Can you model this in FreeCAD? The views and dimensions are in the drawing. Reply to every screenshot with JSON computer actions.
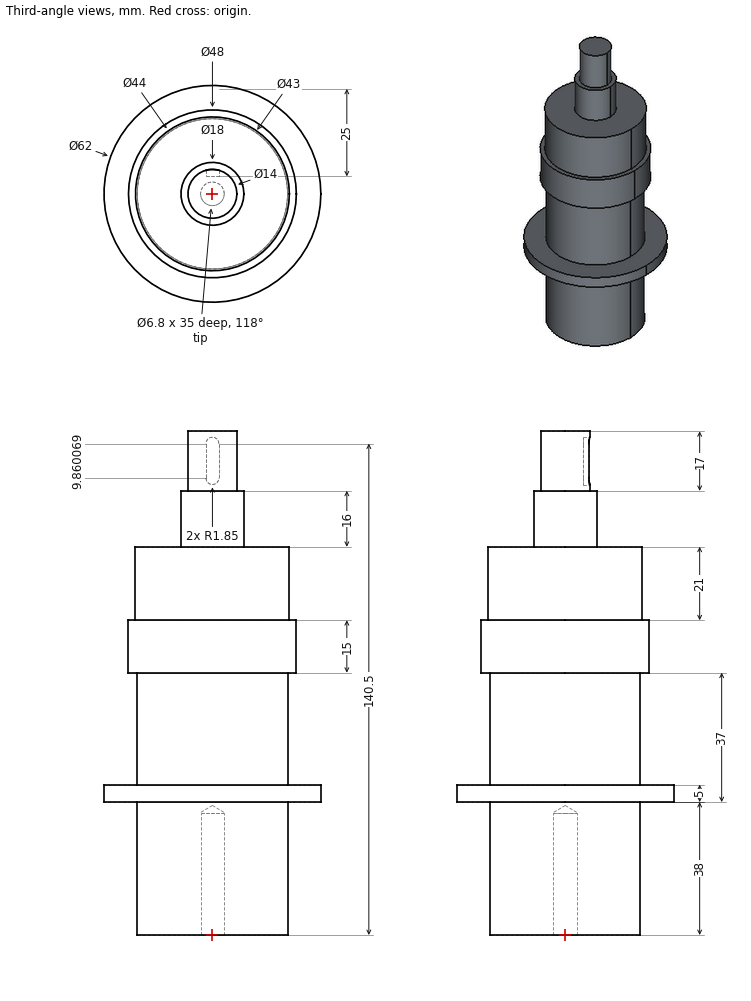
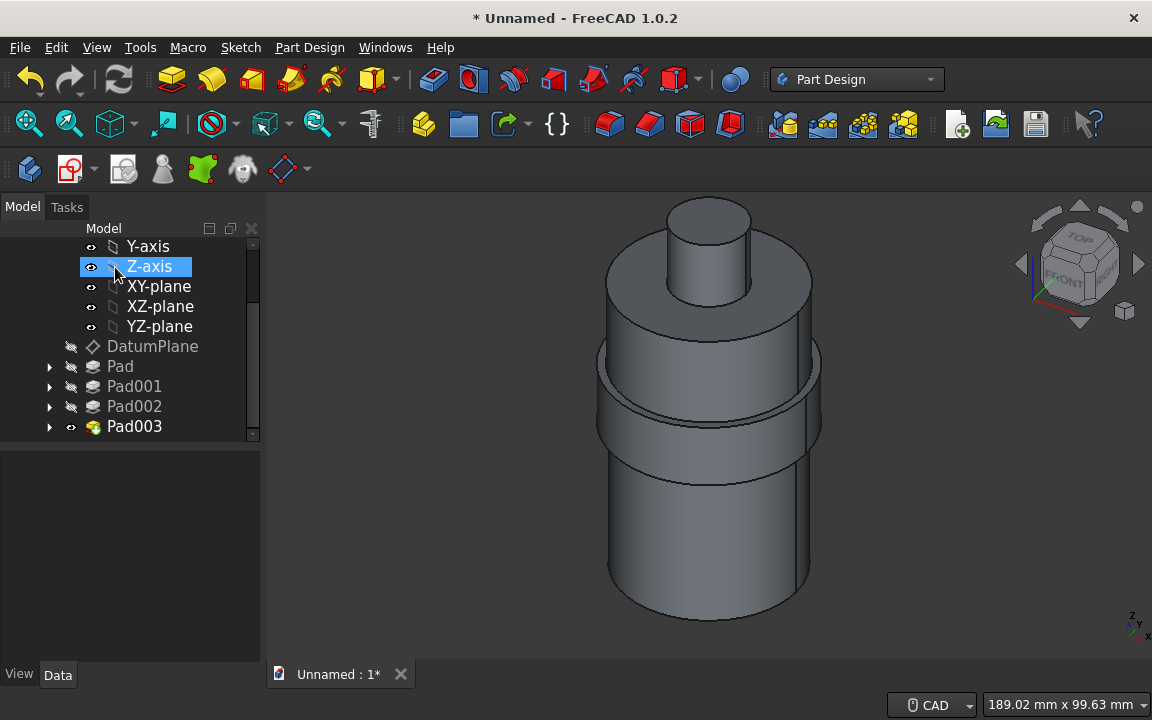
{"action": "left_click", "coordinate": [30, 124]}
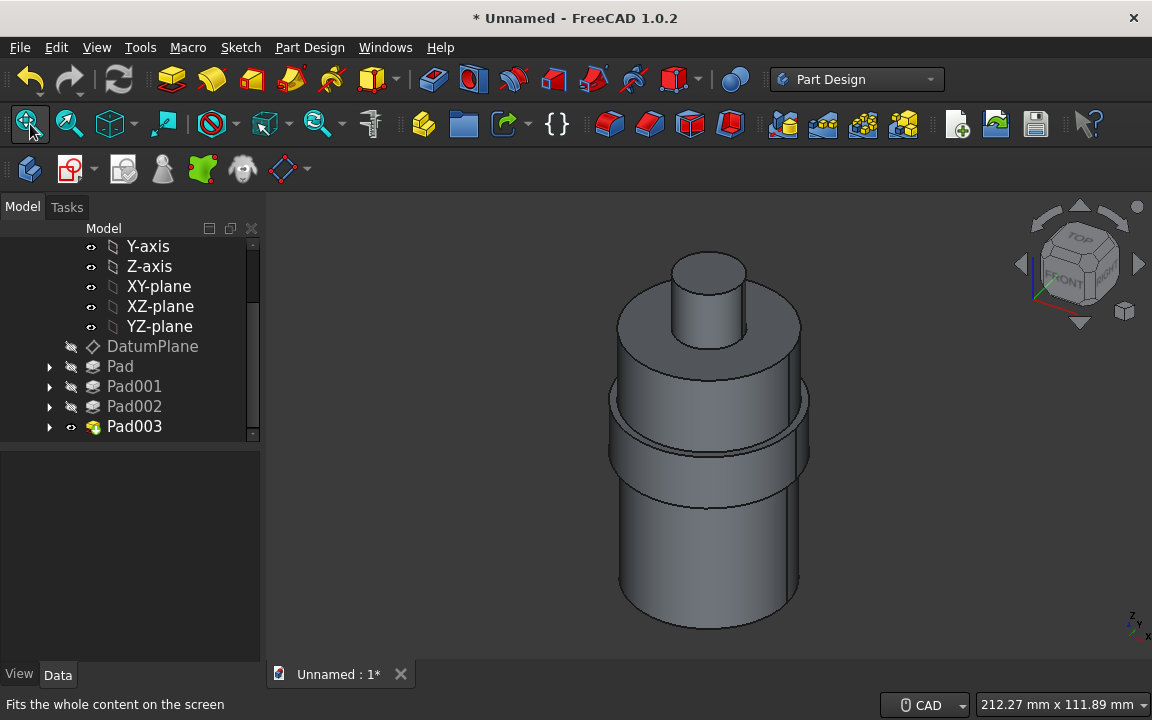
{"action": "left_click", "coordinate": [709, 272]}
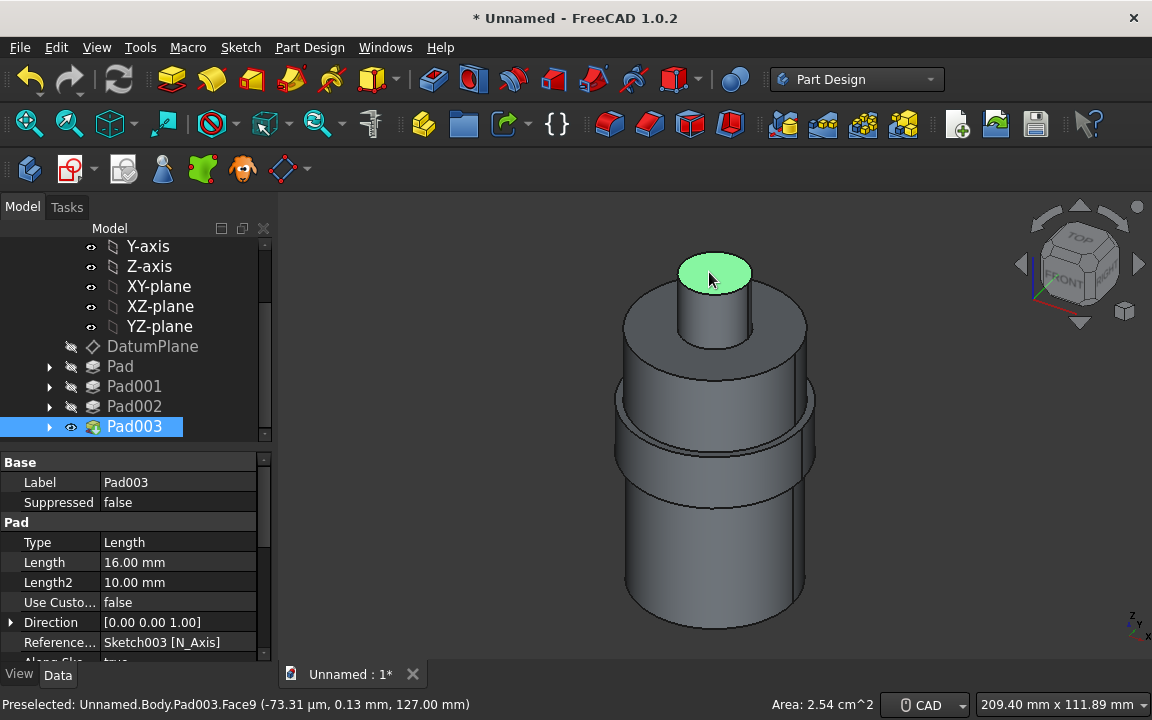
{"action": "left_click", "coordinate": [70, 170]}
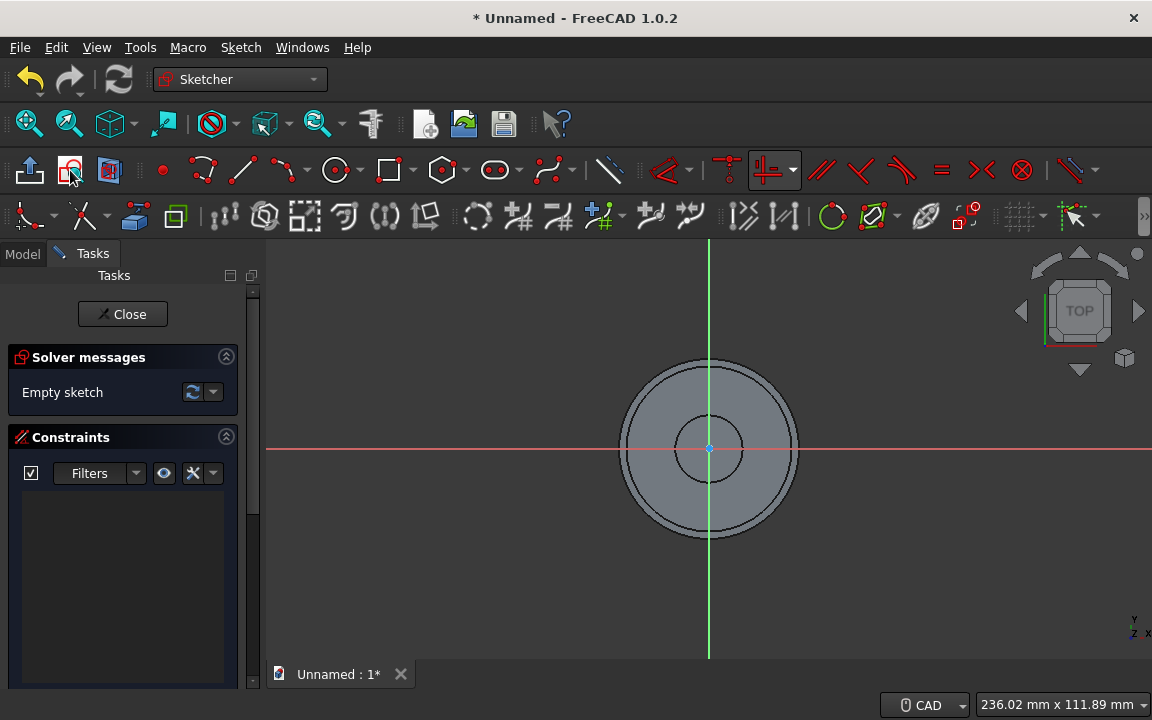
{"action": "scroll", "coordinate": [726, 449], "scroll_direction": "up", "scroll_amount": 8}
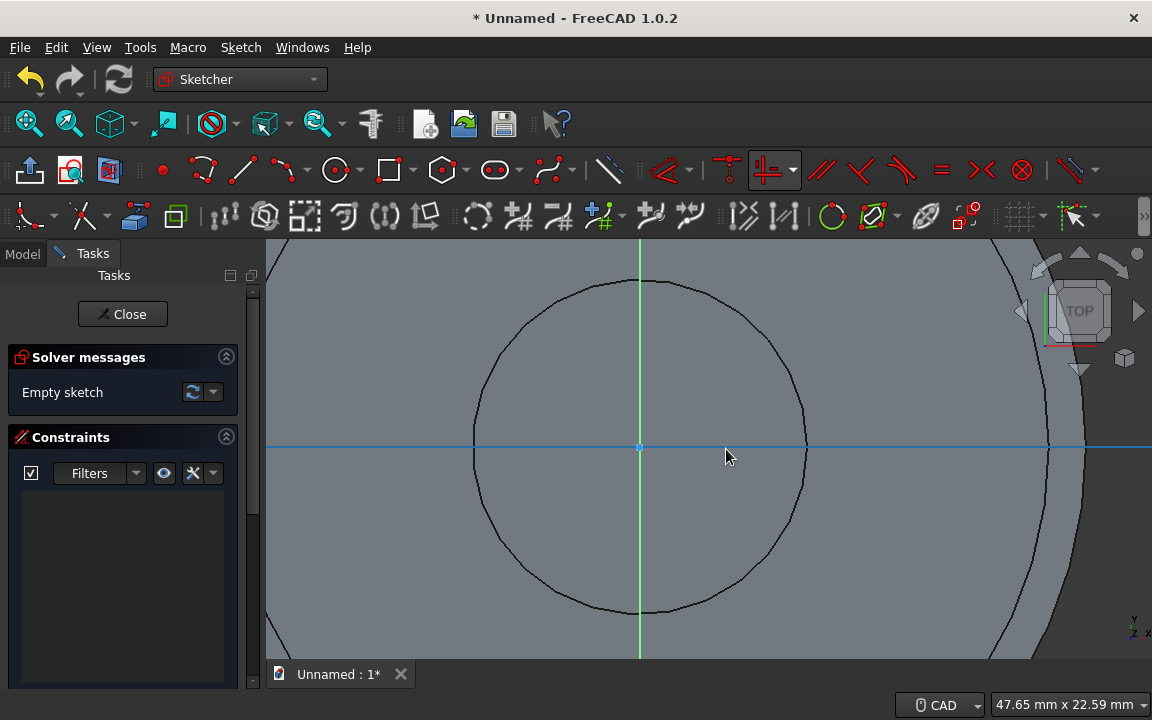
{"action": "key", "text": "g c"}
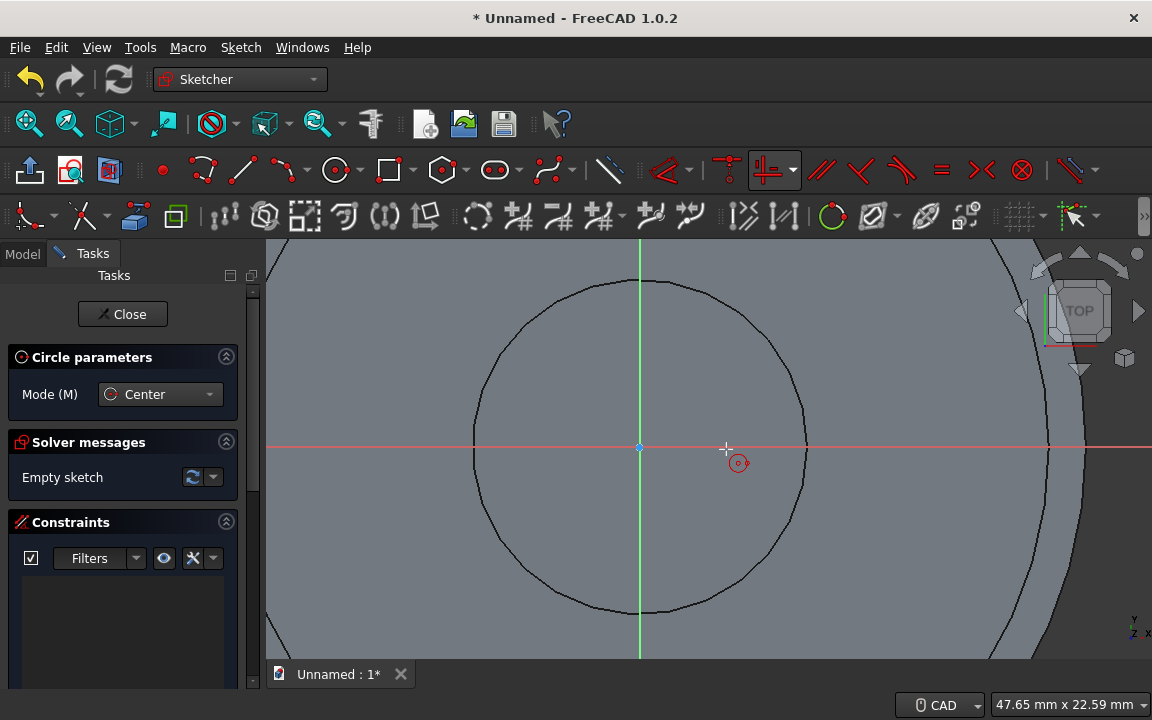
{"action": "left_click", "coordinate": [640, 447]}
{"action": "left_click", "coordinate": [732, 355]}
{"action": "key", "text": "Escape"}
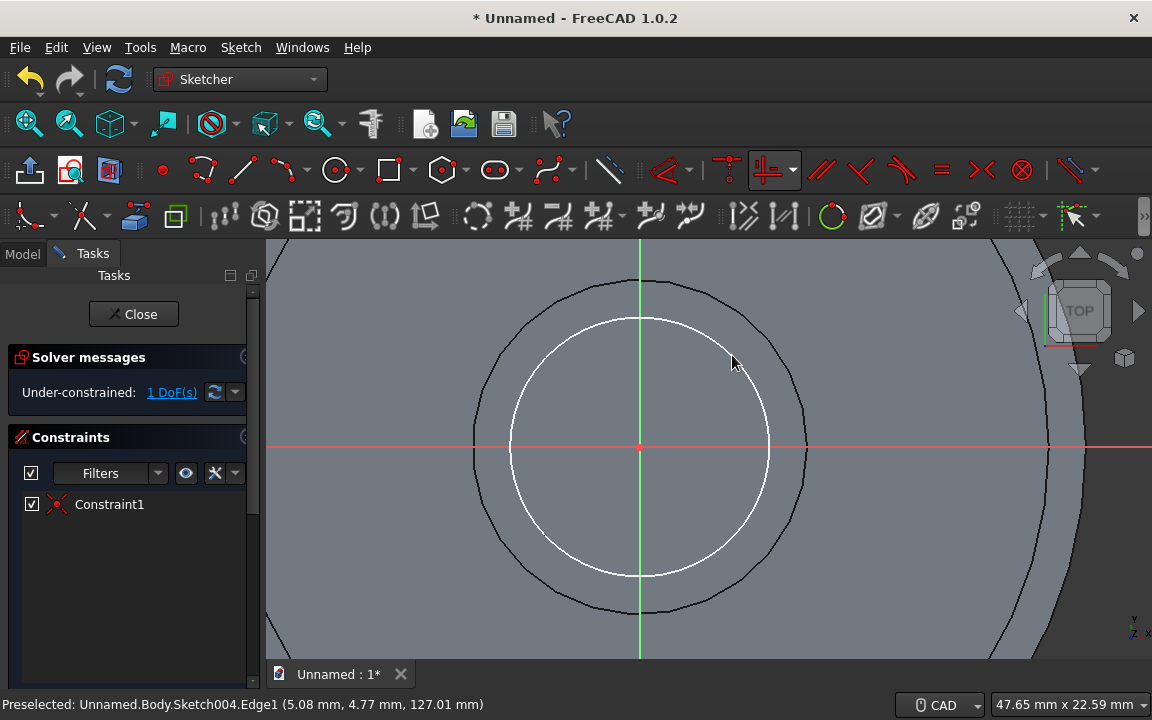
{"action": "left_click", "coordinate": [664, 170]}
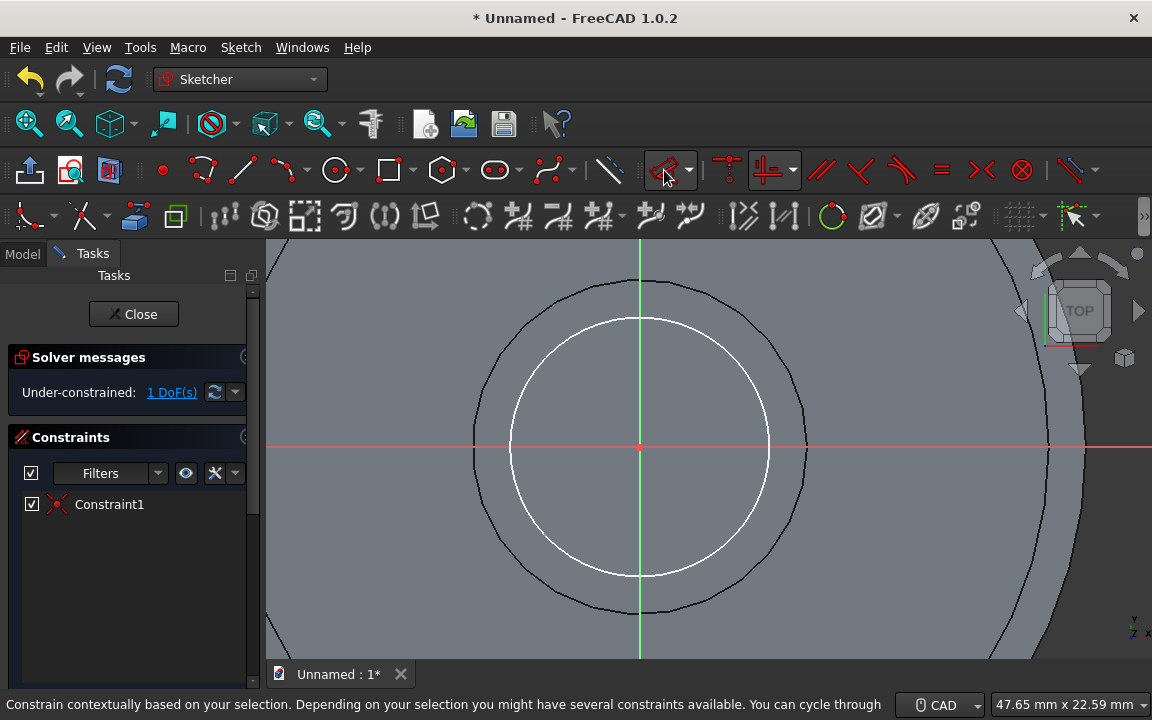
{"action": "left_click", "coordinate": [731, 355]}
{"action": "left_click", "coordinate": [754, 332]}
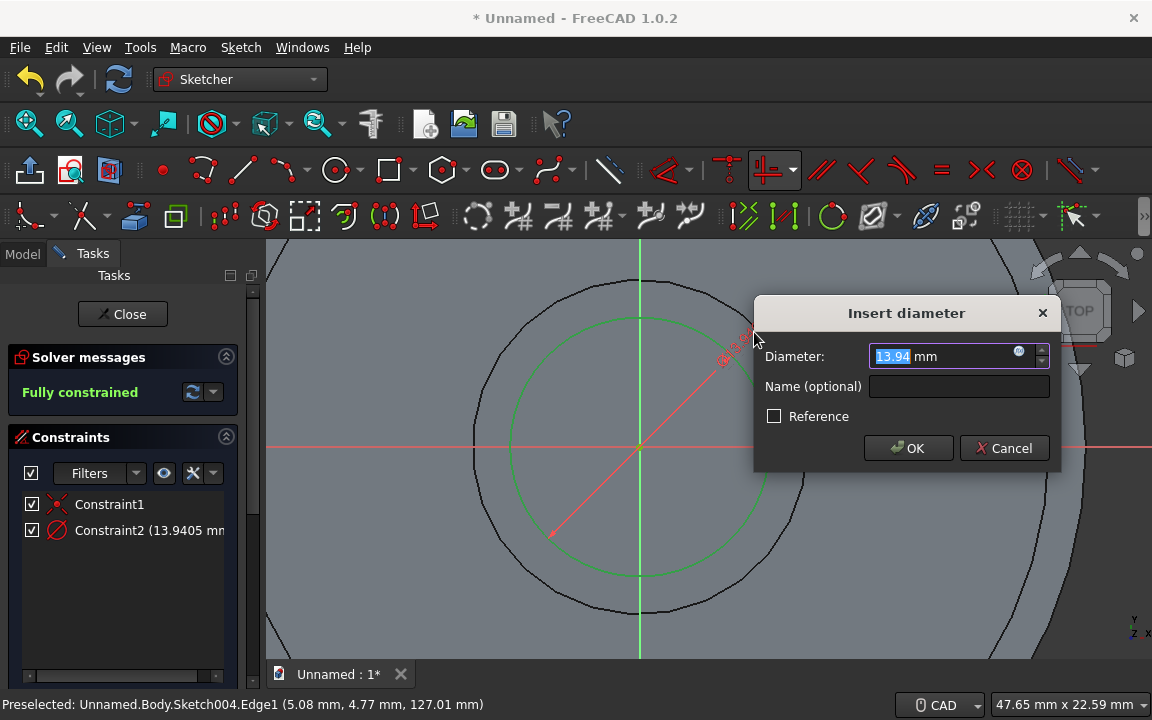
{"action": "type", "text": "14"}
{"action": "key", "text": "Return"}
{"action": "key", "text": "Escape"}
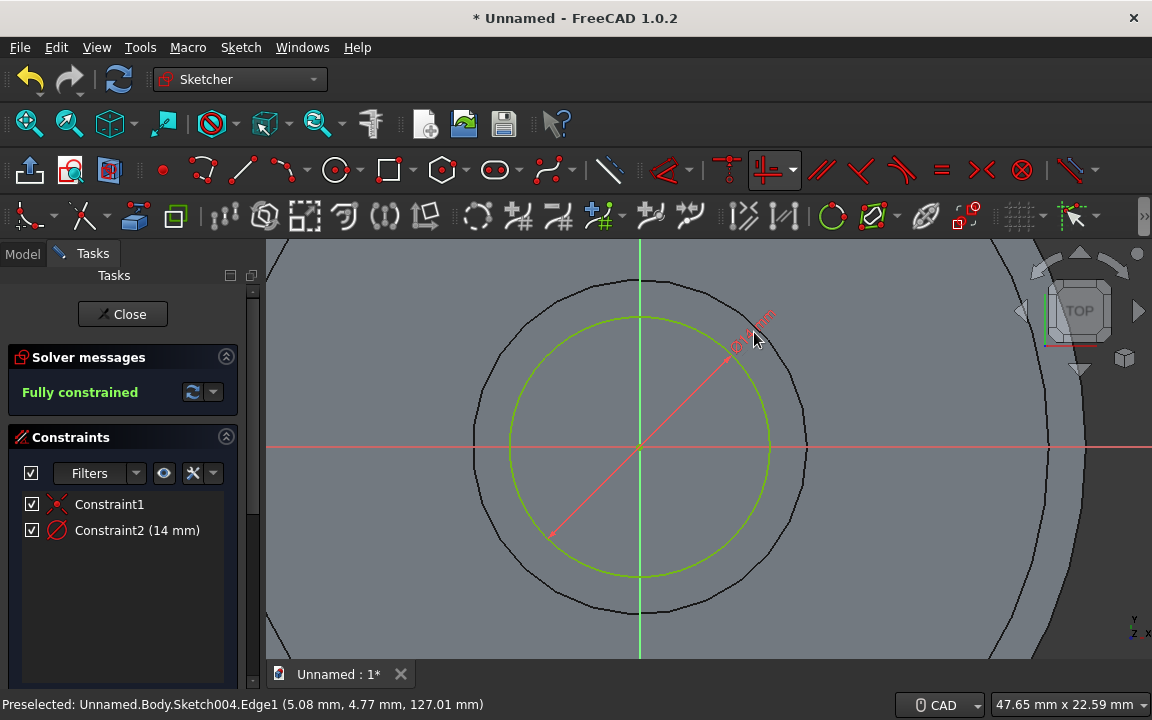
{"action": "left_click", "coordinate": [123, 314]}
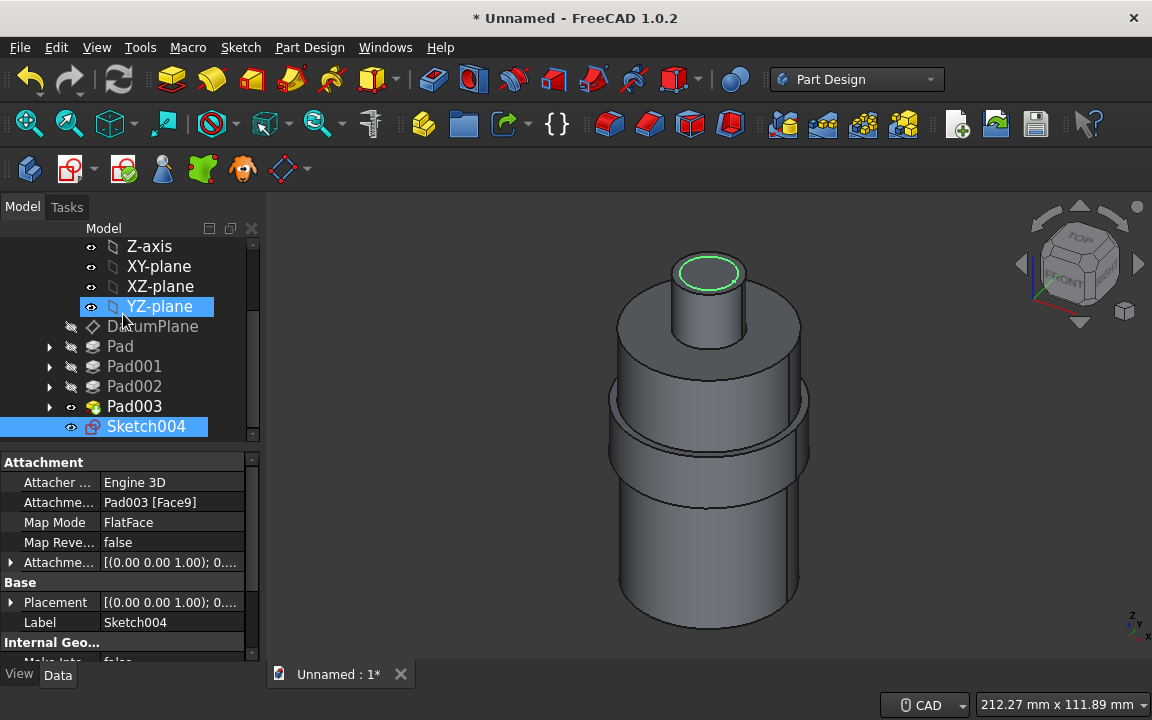
{"action": "left_click", "coordinate": [172, 80]}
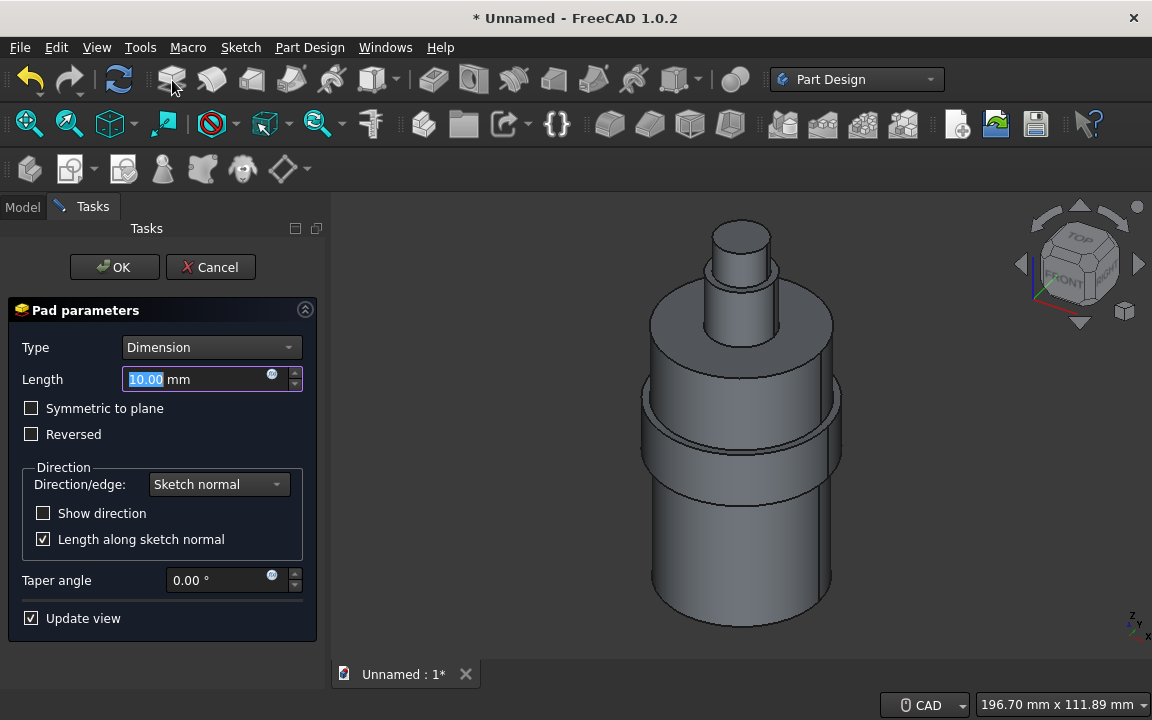
{"action": "type", "text": "17"}
{"action": "key", "text": "Tab"}